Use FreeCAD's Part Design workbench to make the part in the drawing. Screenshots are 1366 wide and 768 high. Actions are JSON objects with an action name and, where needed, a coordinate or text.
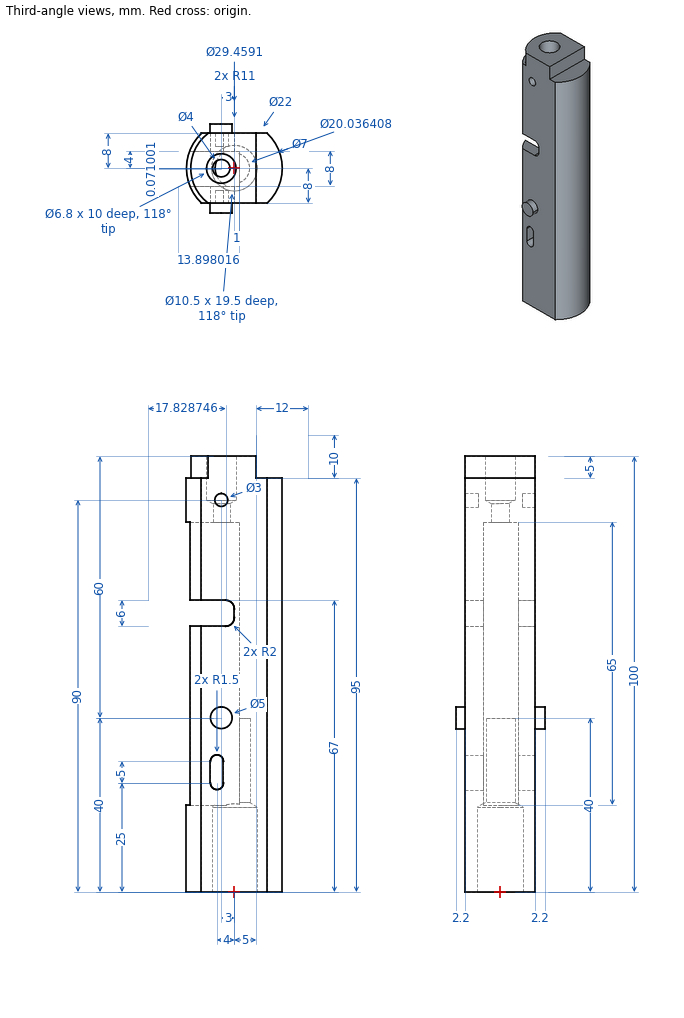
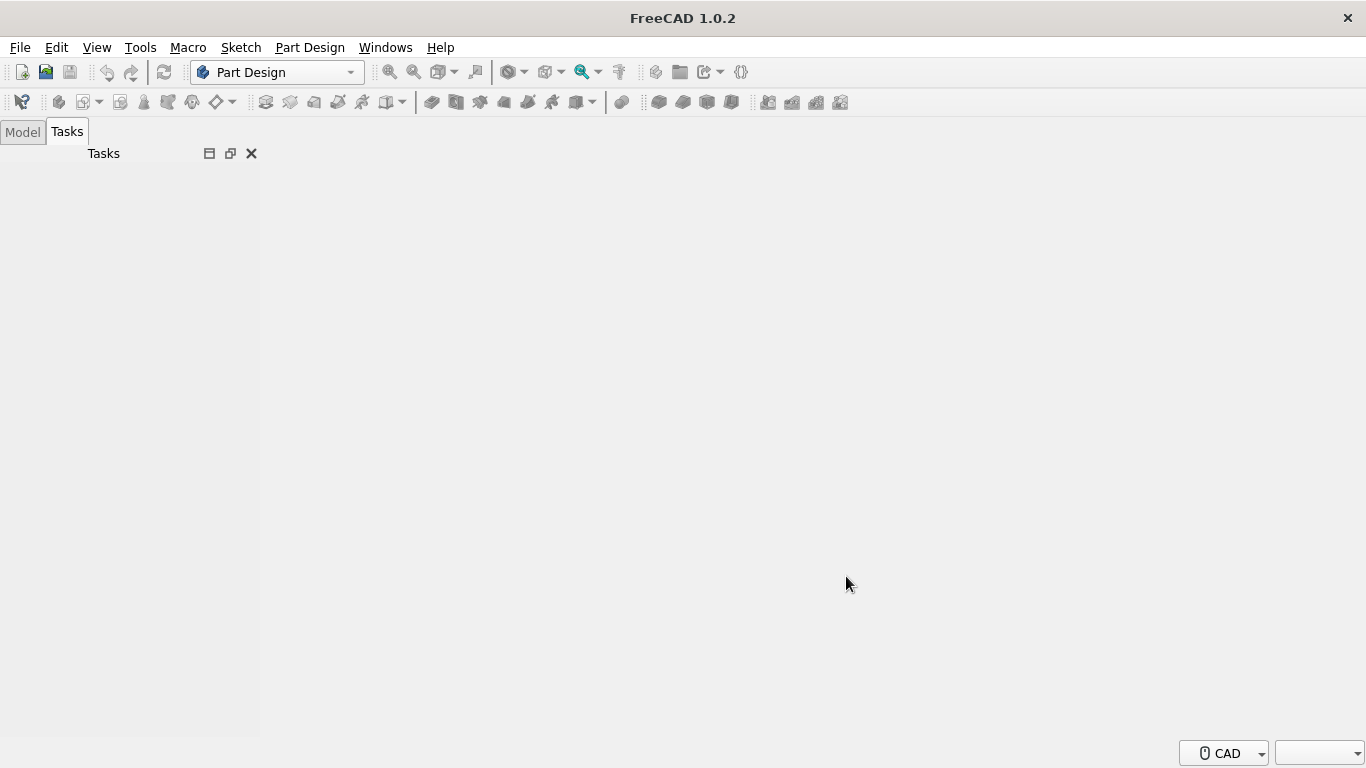
{"action": "key", "text": "ctrl+n"}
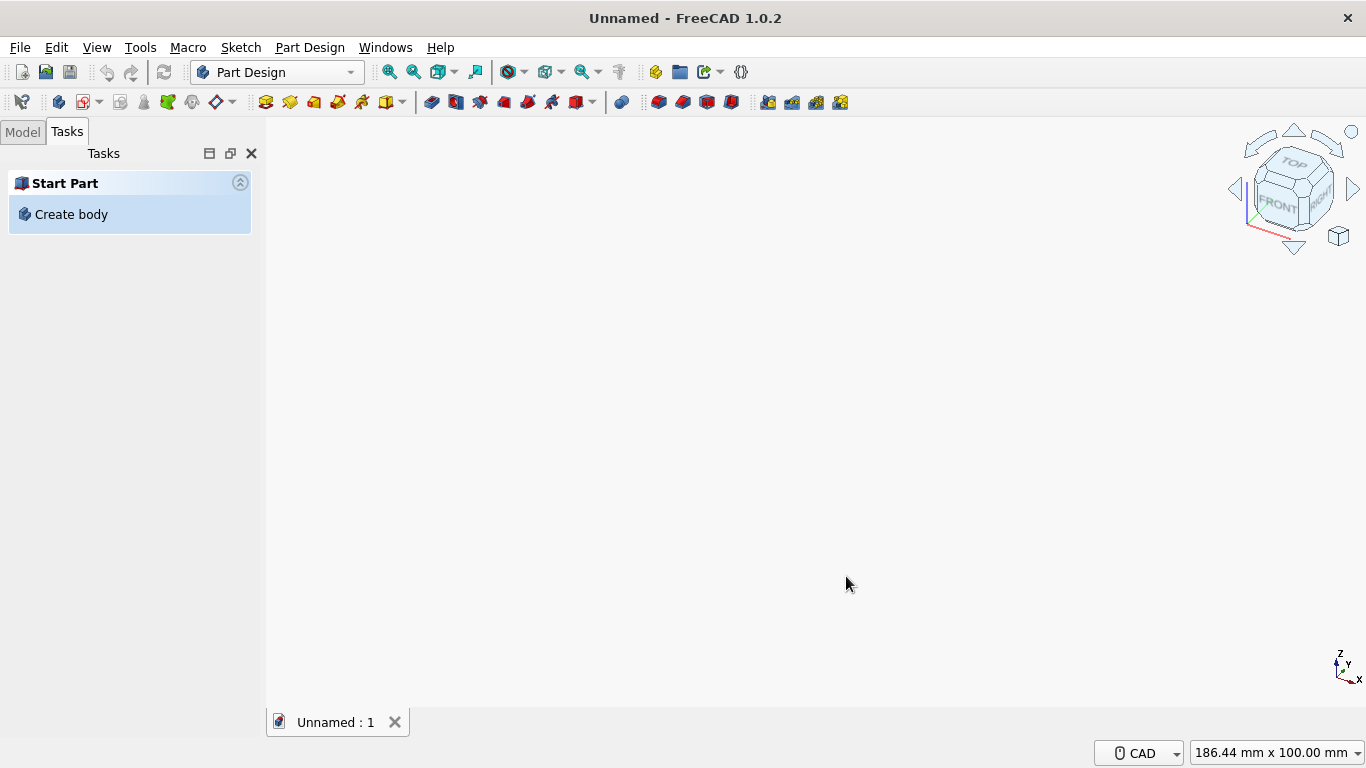
{"action": "left_click", "coordinate": [84, 102]}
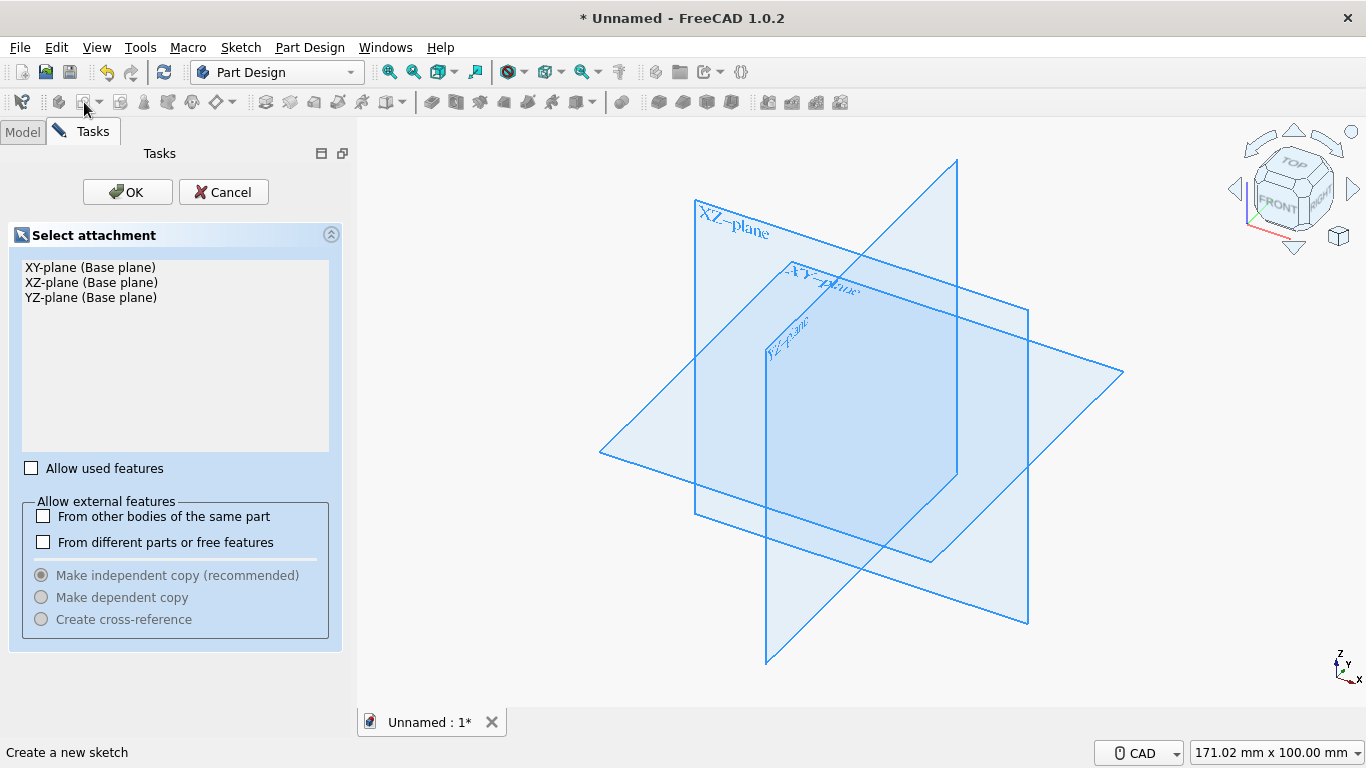
{"action": "left_click", "coordinate": [82, 268]}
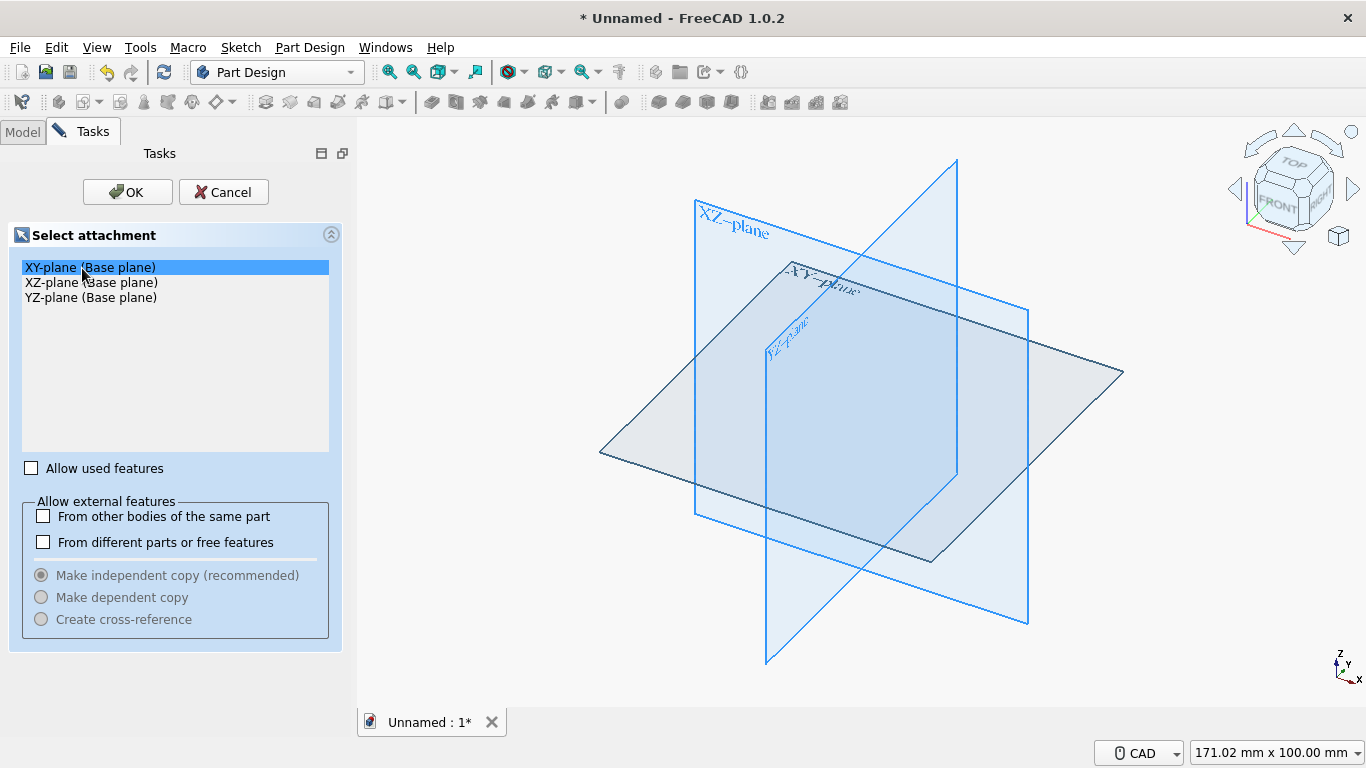
{"action": "left_click", "coordinate": [128, 192]}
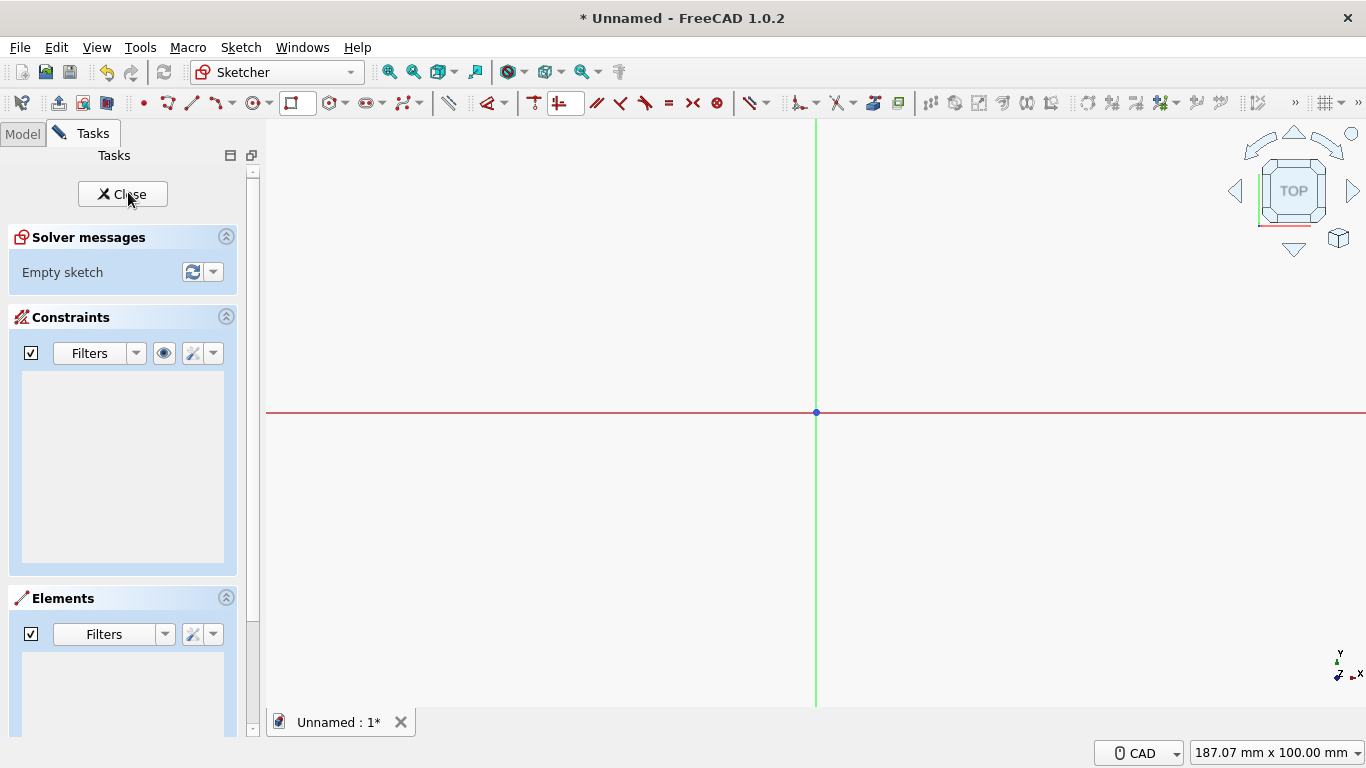
{"action": "scroll", "coordinate": [856, 413], "scroll_direction": "up", "scroll_amount": 5}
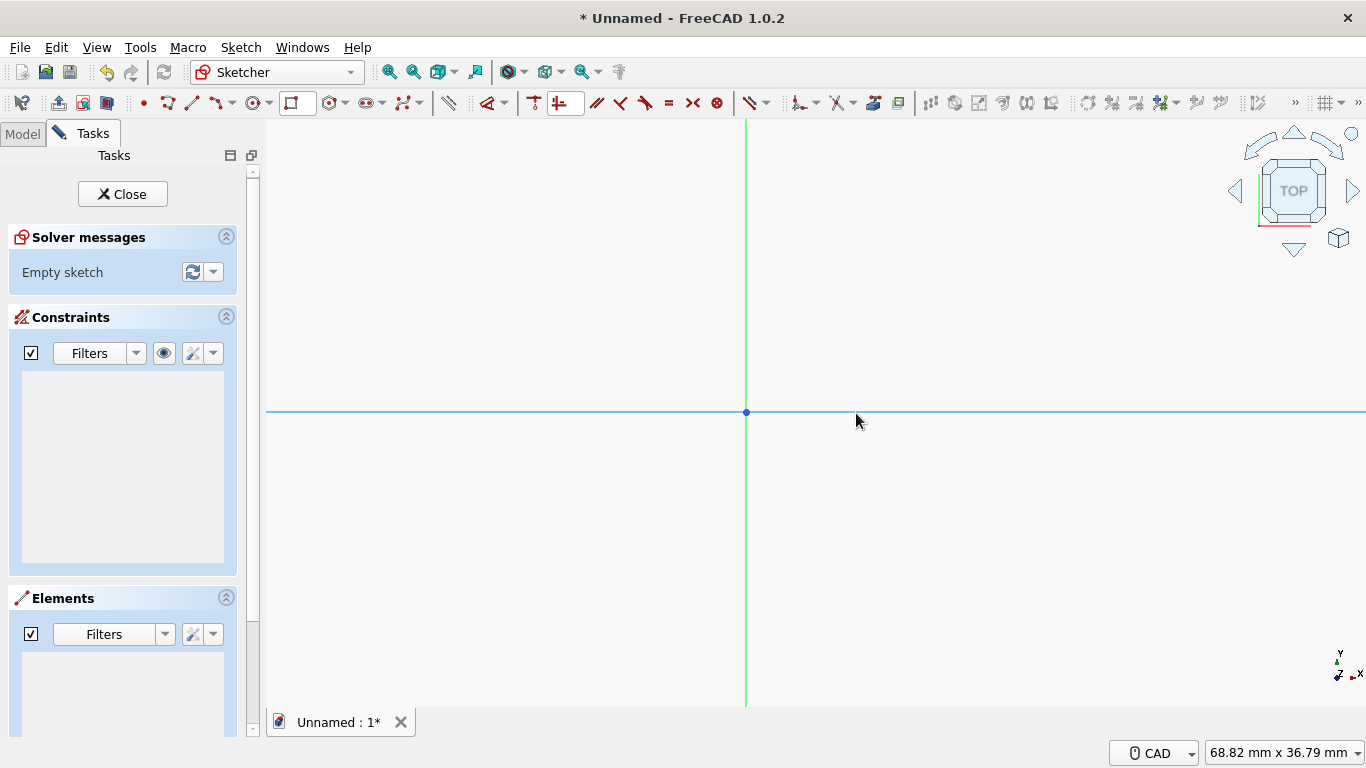
{"action": "key", "text": "g c"}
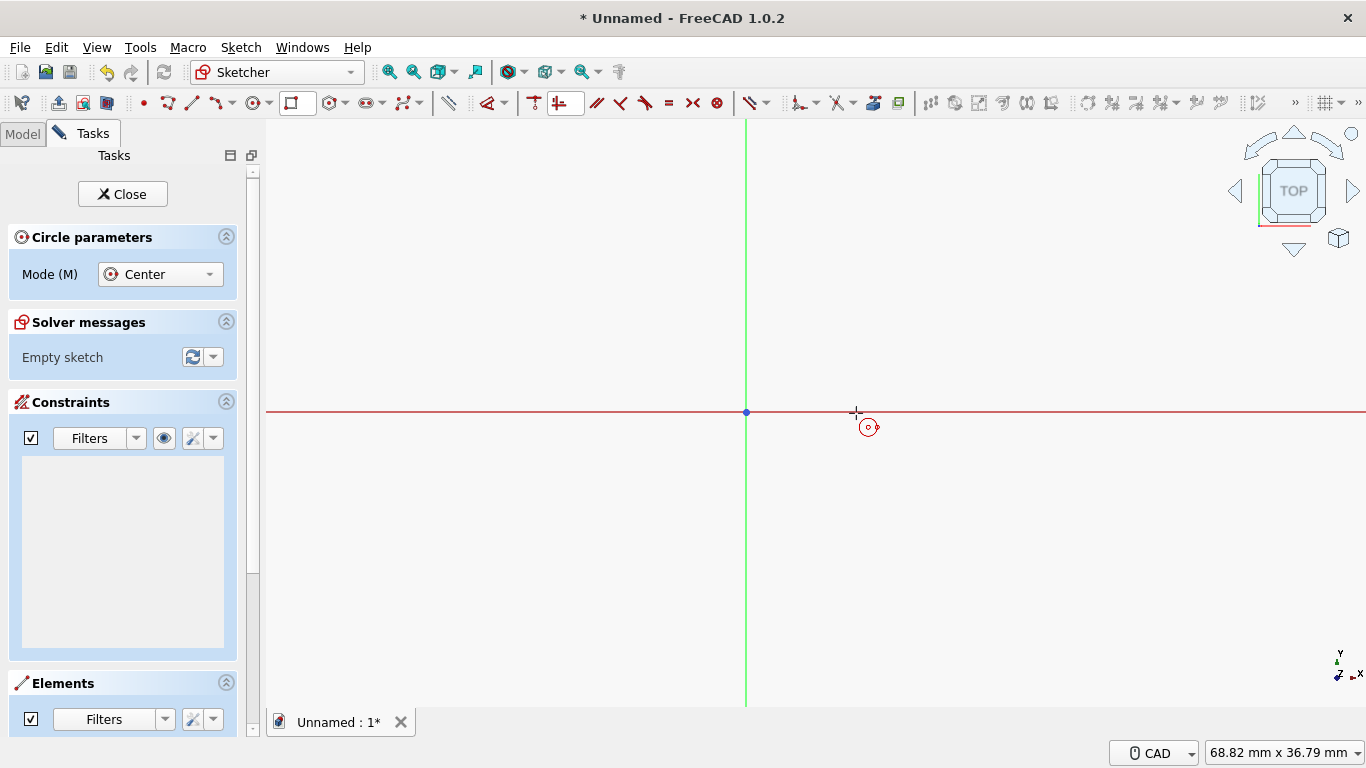
{"action": "left_click", "coordinate": [746, 412]}
{"action": "mouse_move", "coordinate": [871, 288]}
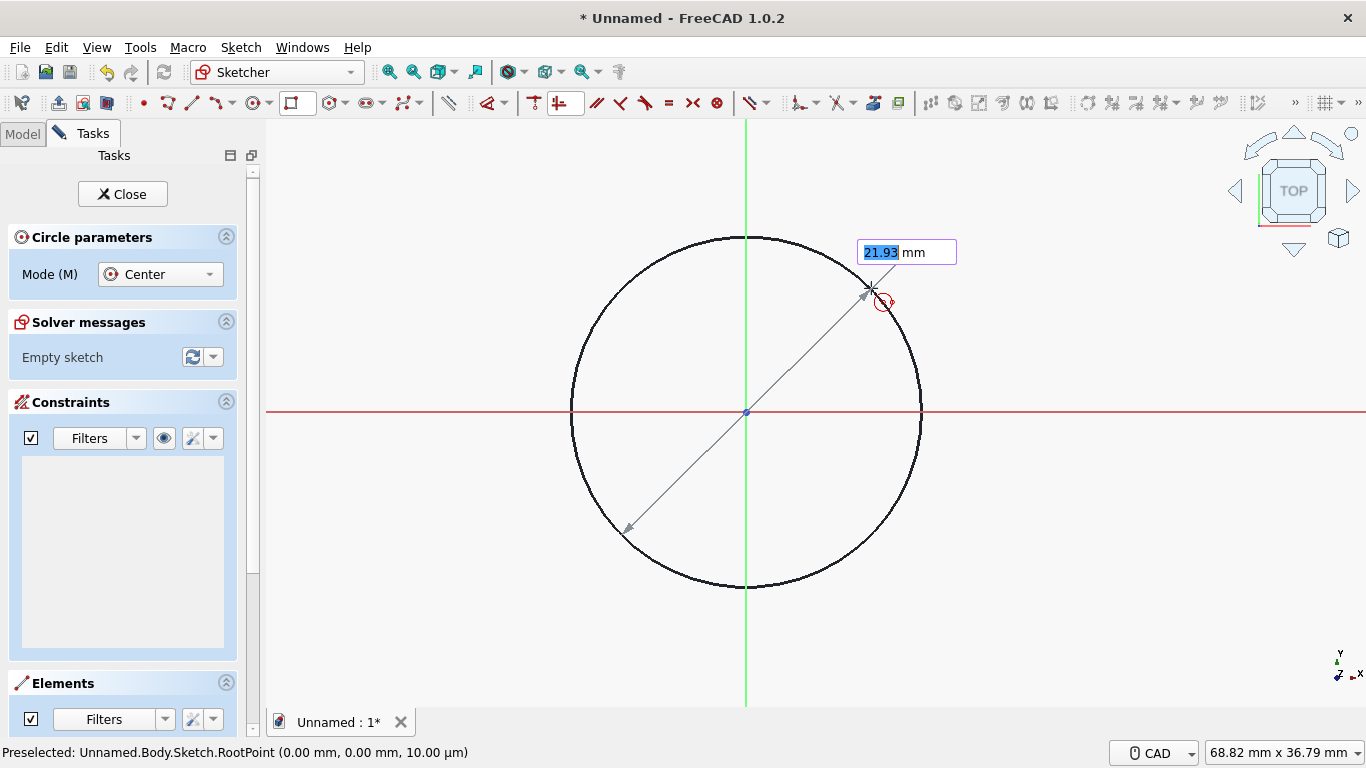
{"action": "type", "text": "22"}
{"action": "key", "text": "Return"}
{"action": "key", "text": "Escape"}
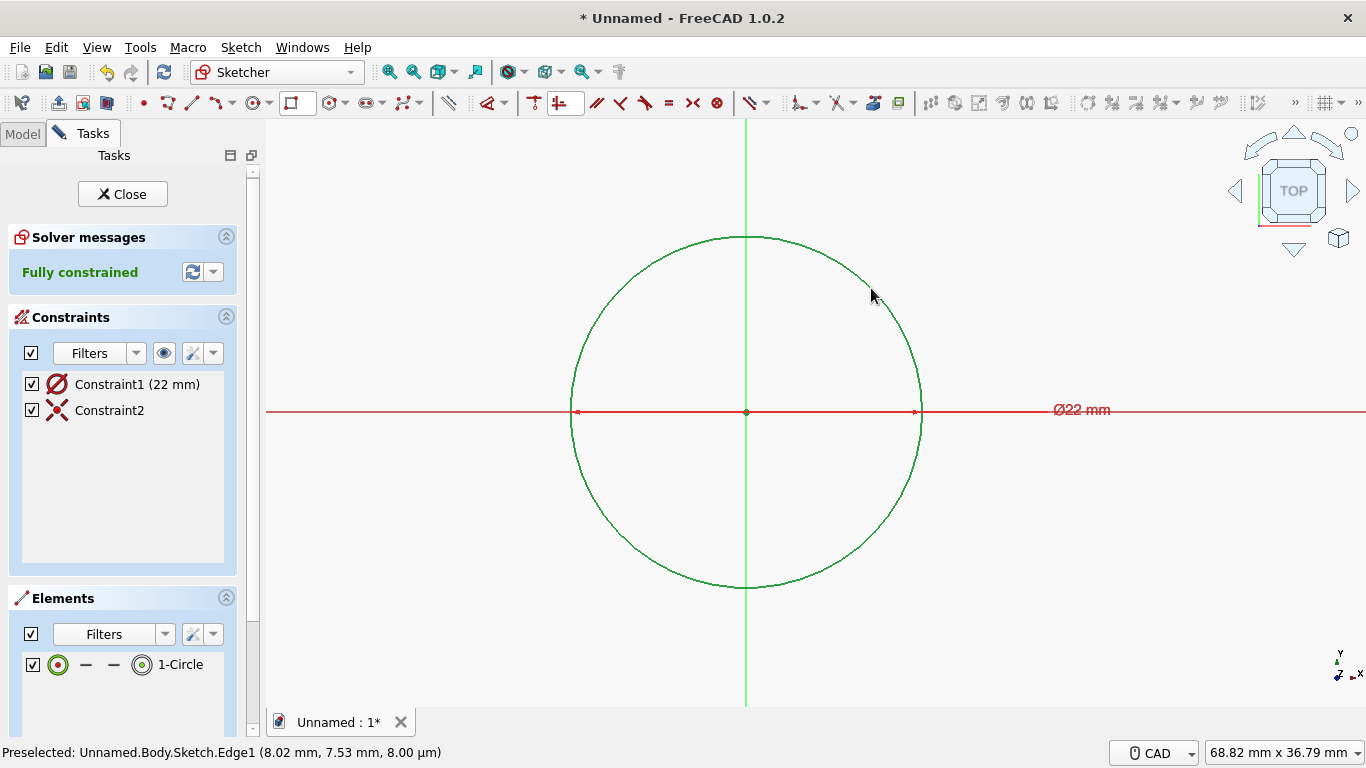
{"action": "left_click", "coordinate": [123, 194]}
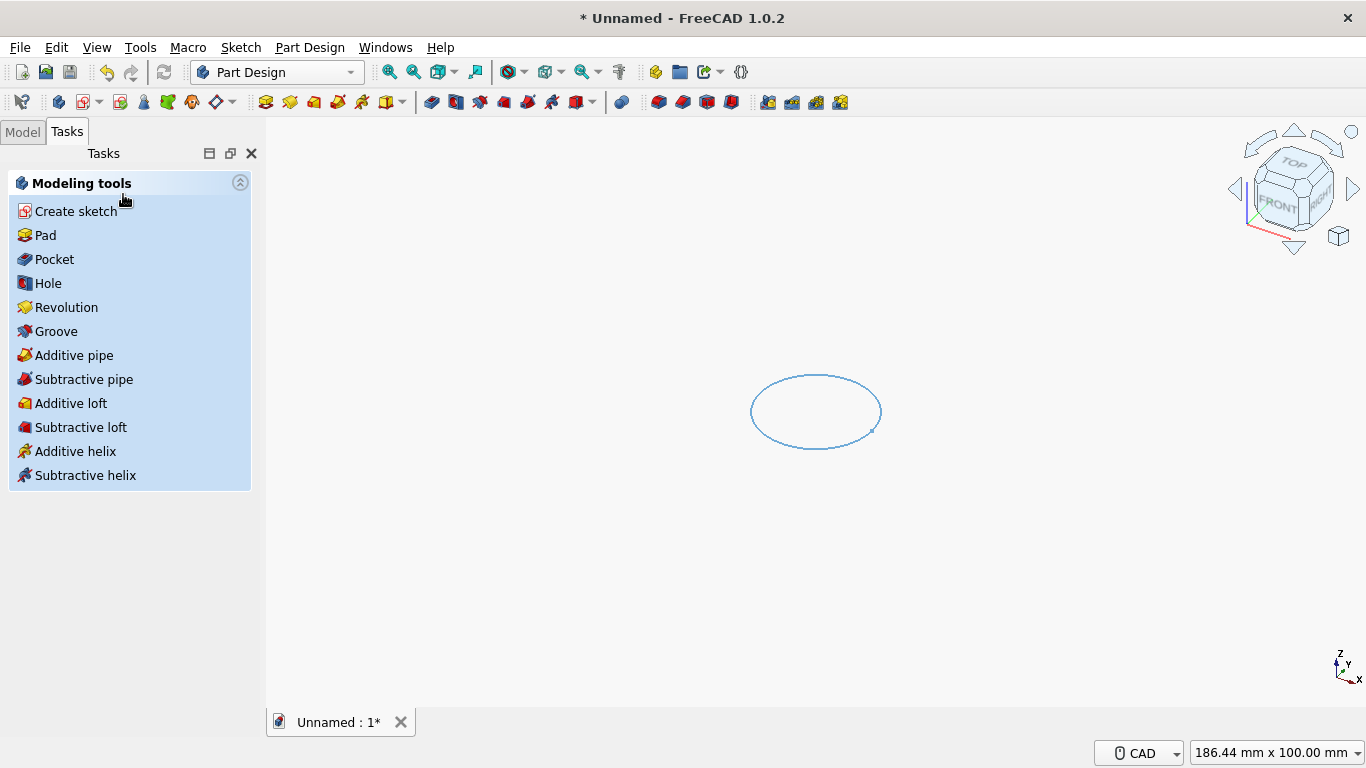
{"action": "left_click", "coordinate": [266, 102]}